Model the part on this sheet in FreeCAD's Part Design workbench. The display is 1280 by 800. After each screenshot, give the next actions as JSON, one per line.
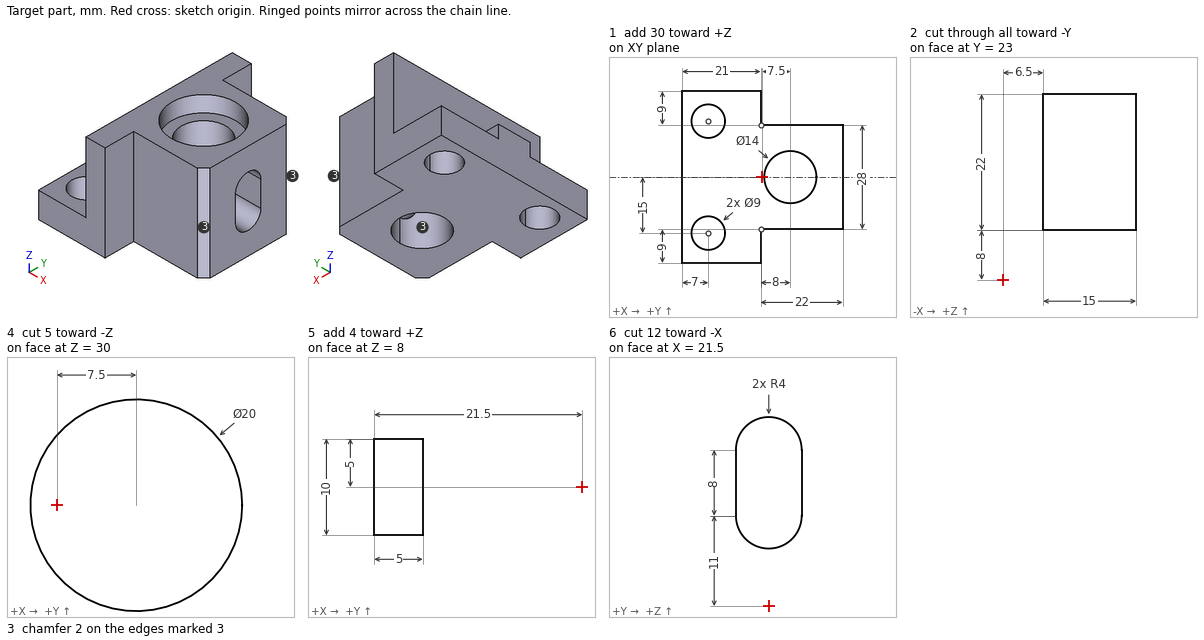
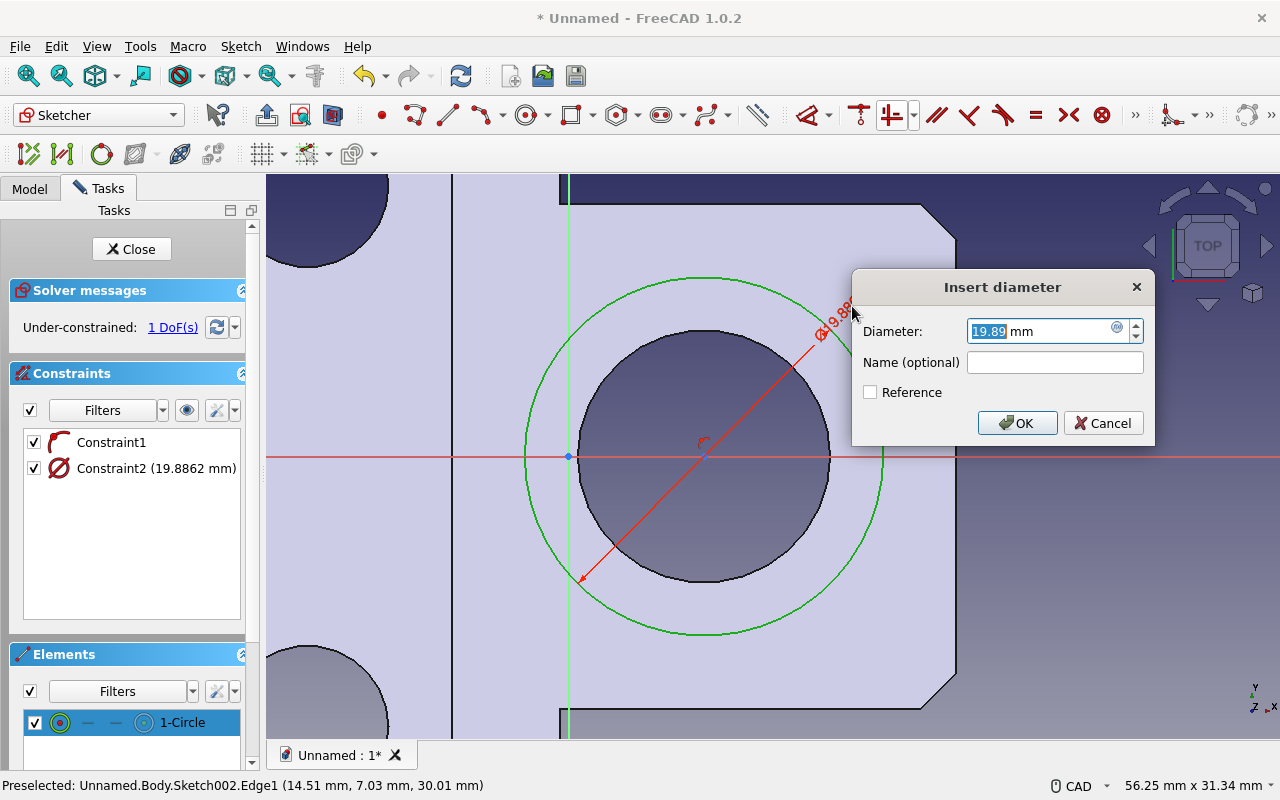
{"action": "type", "text": "20"}
{"action": "key", "text": "Return"}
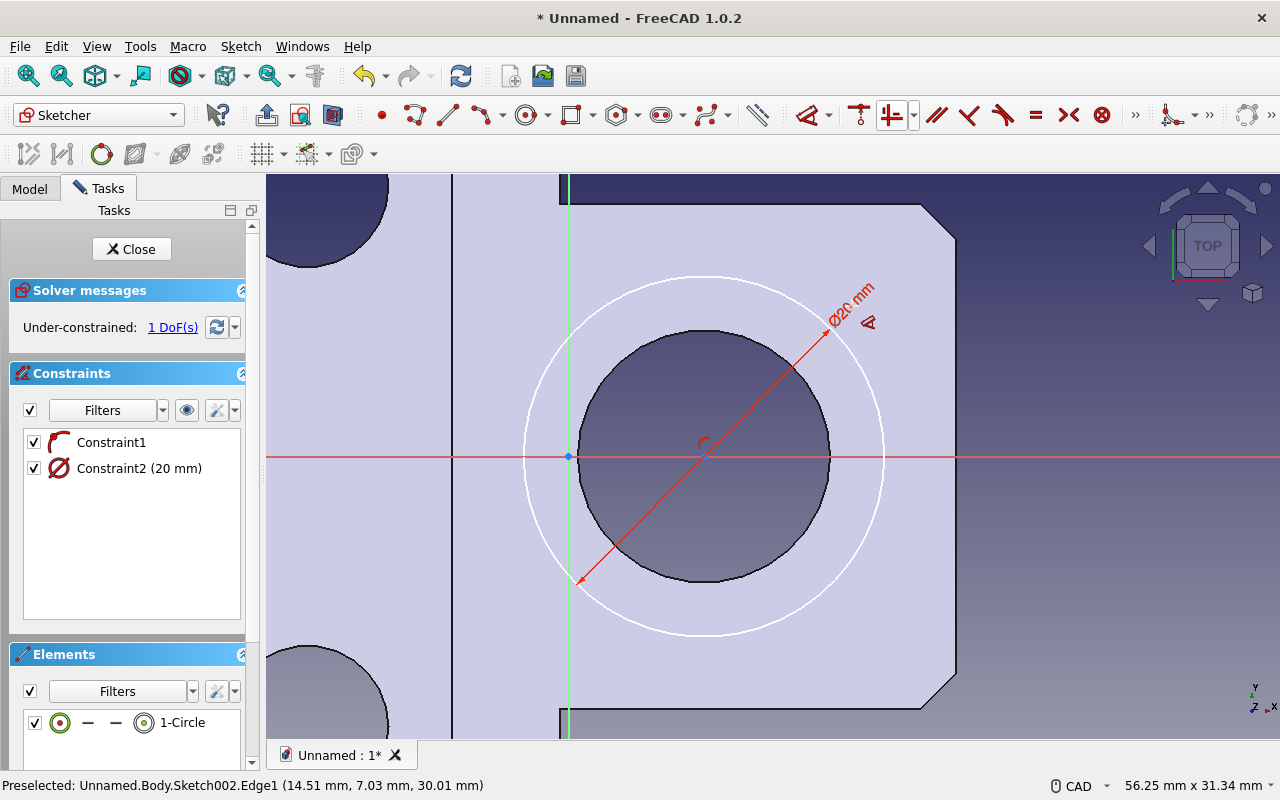
{"action": "left_click", "coordinate": [704, 456]}
{"action": "left_click", "coordinate": [636, 490]}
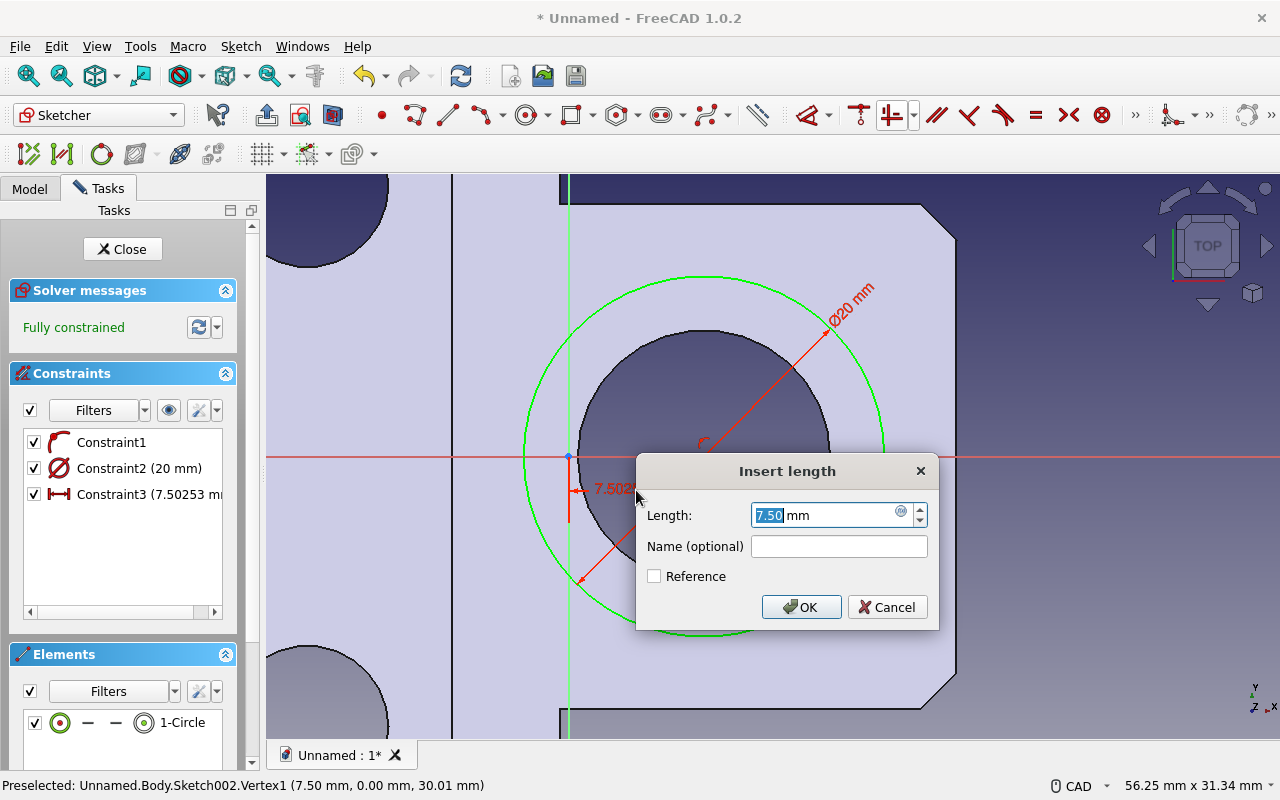
{"action": "type", "text": "7.5"}
{"action": "key", "text": "Return"}
{"action": "key", "text": "Escape"}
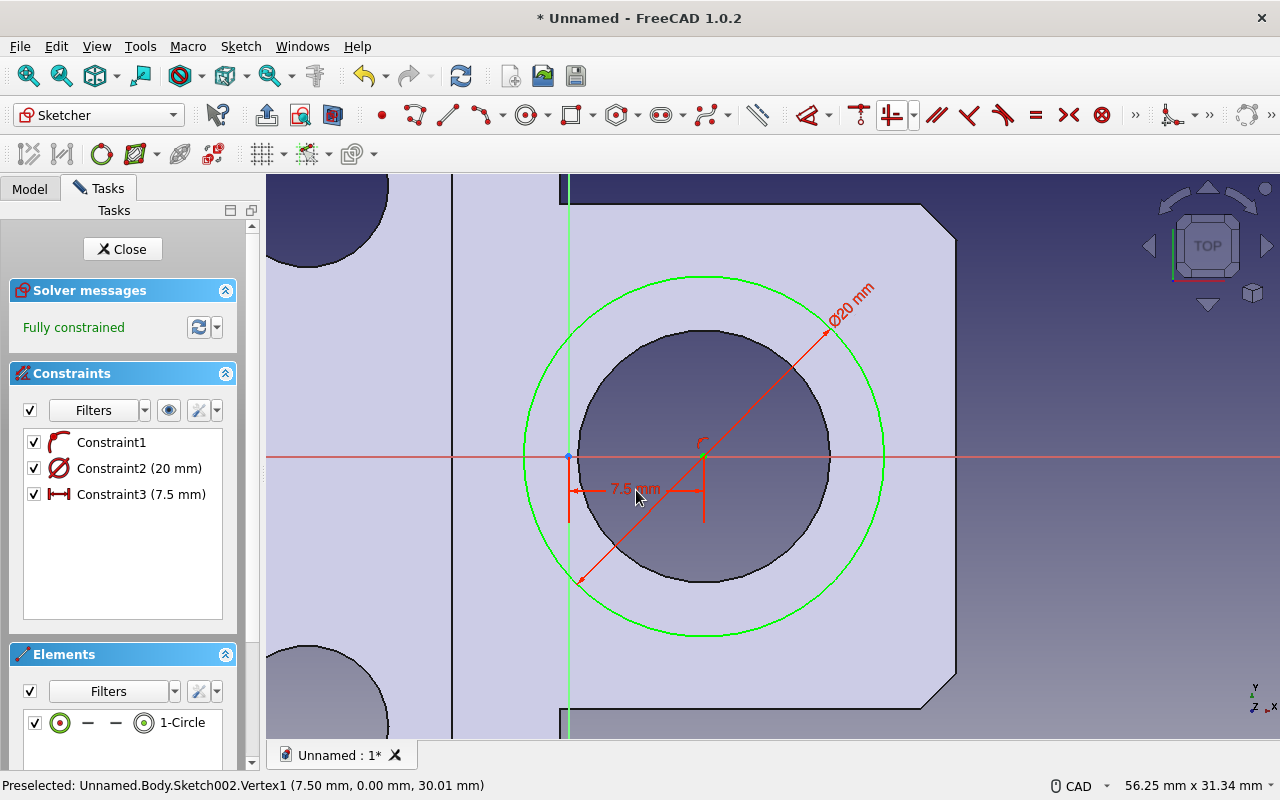
{"action": "left_click", "coordinate": [123, 249]}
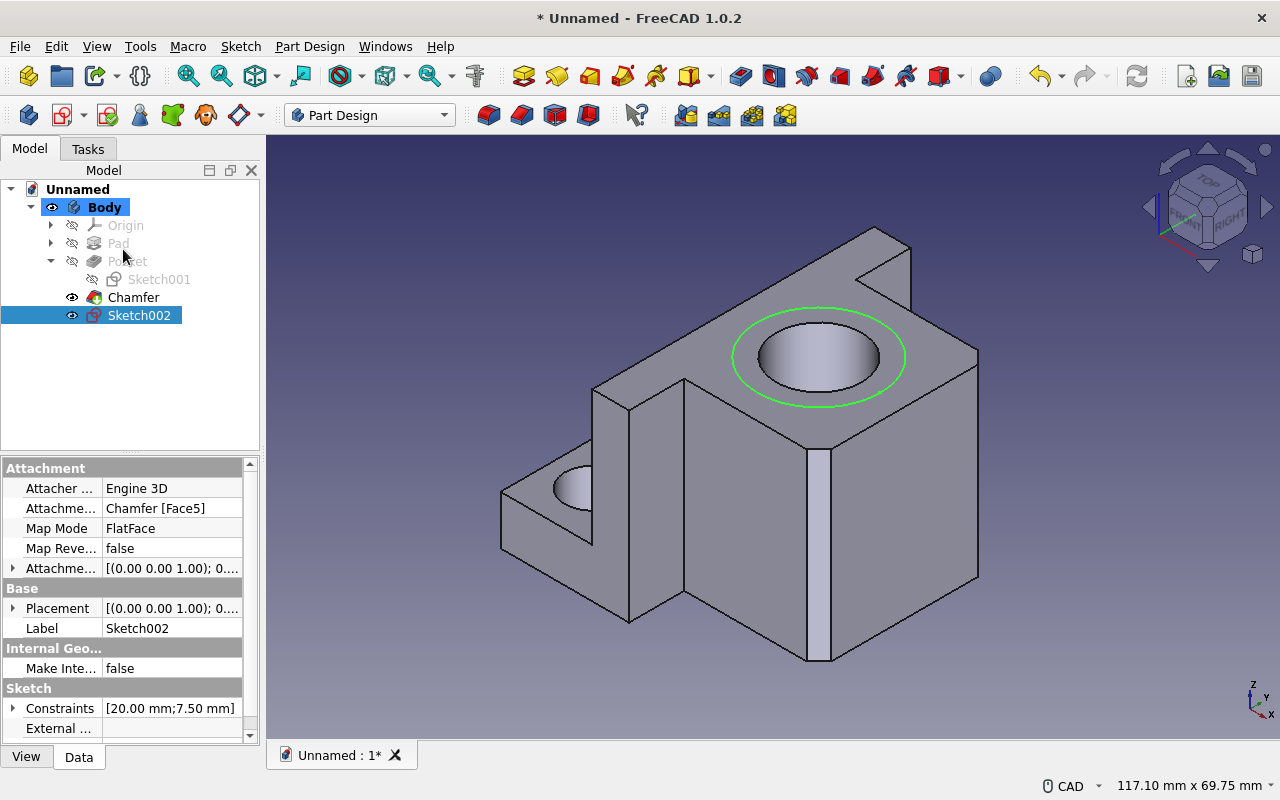
{"action": "left_click", "coordinate": [741, 76]}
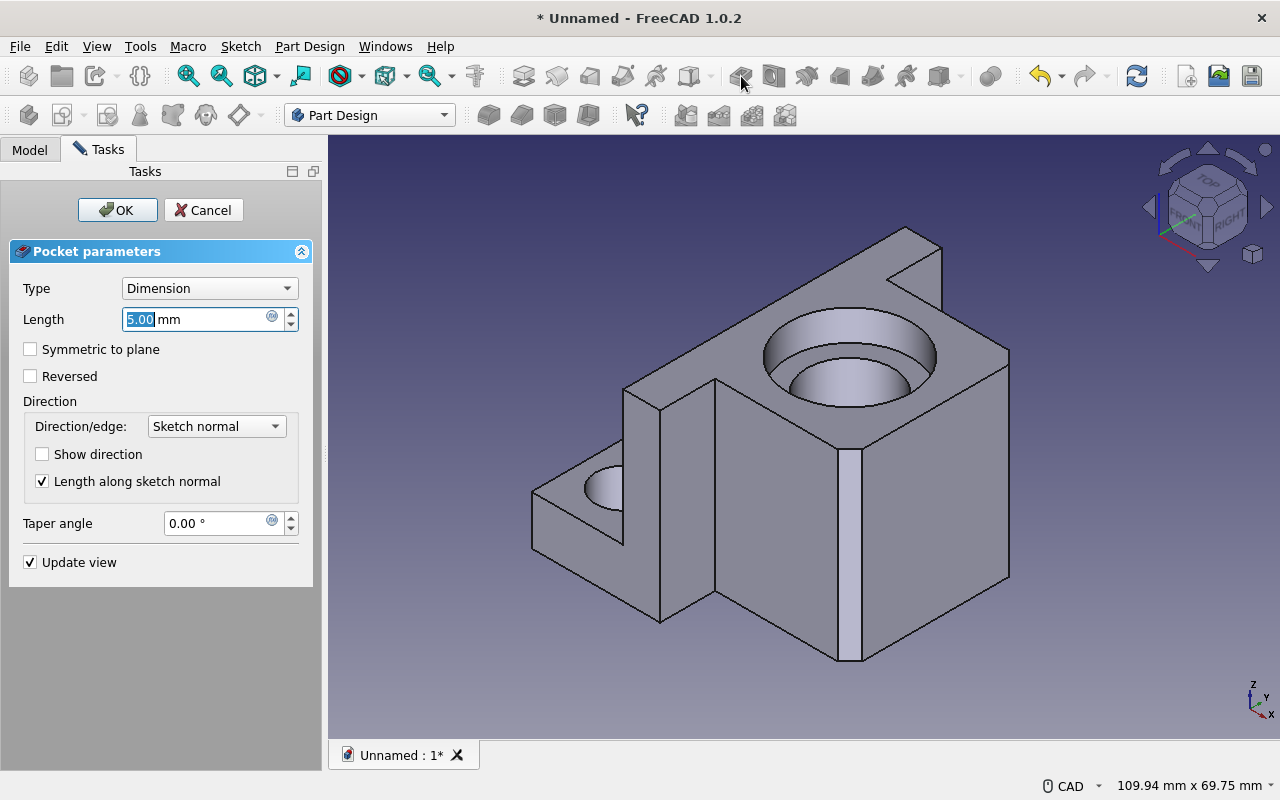
{"action": "type", "text": "5"}
{"action": "key", "text": "Tab"}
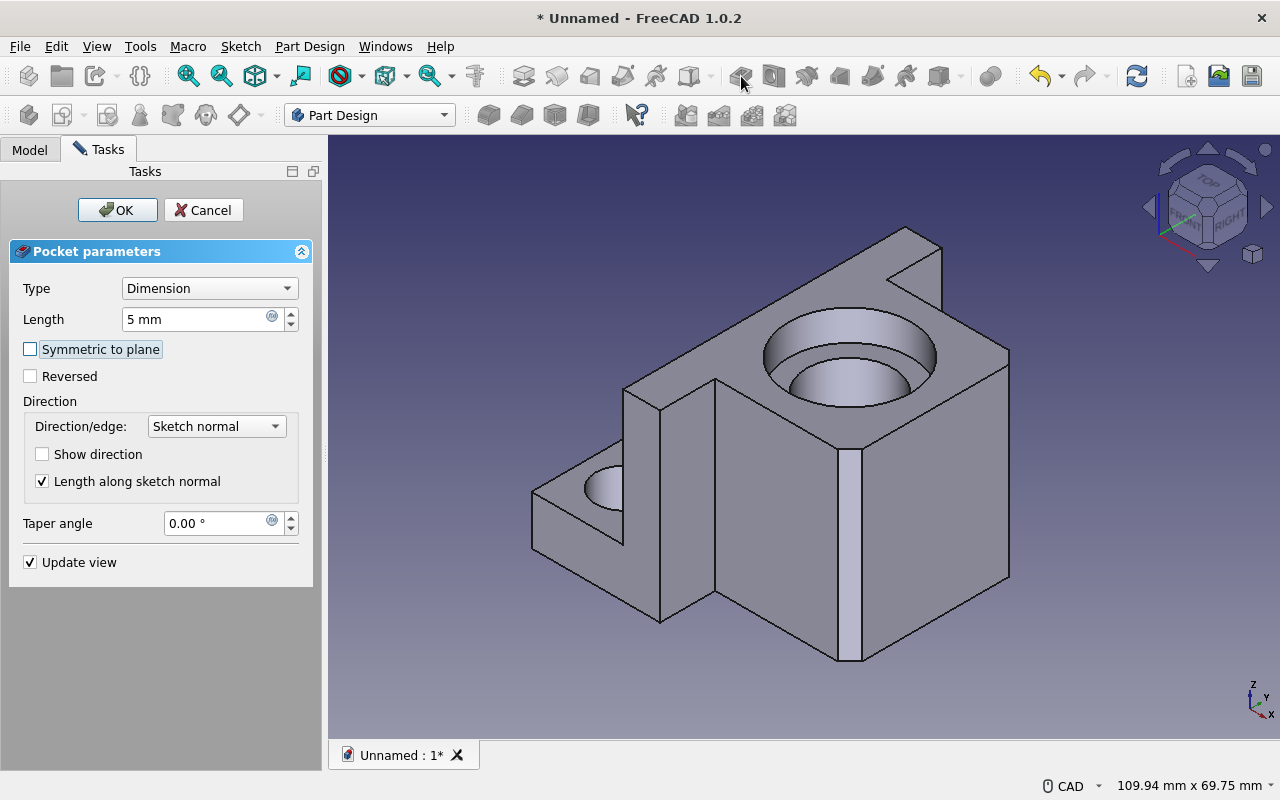
{"action": "left_click", "coordinate": [118, 210]}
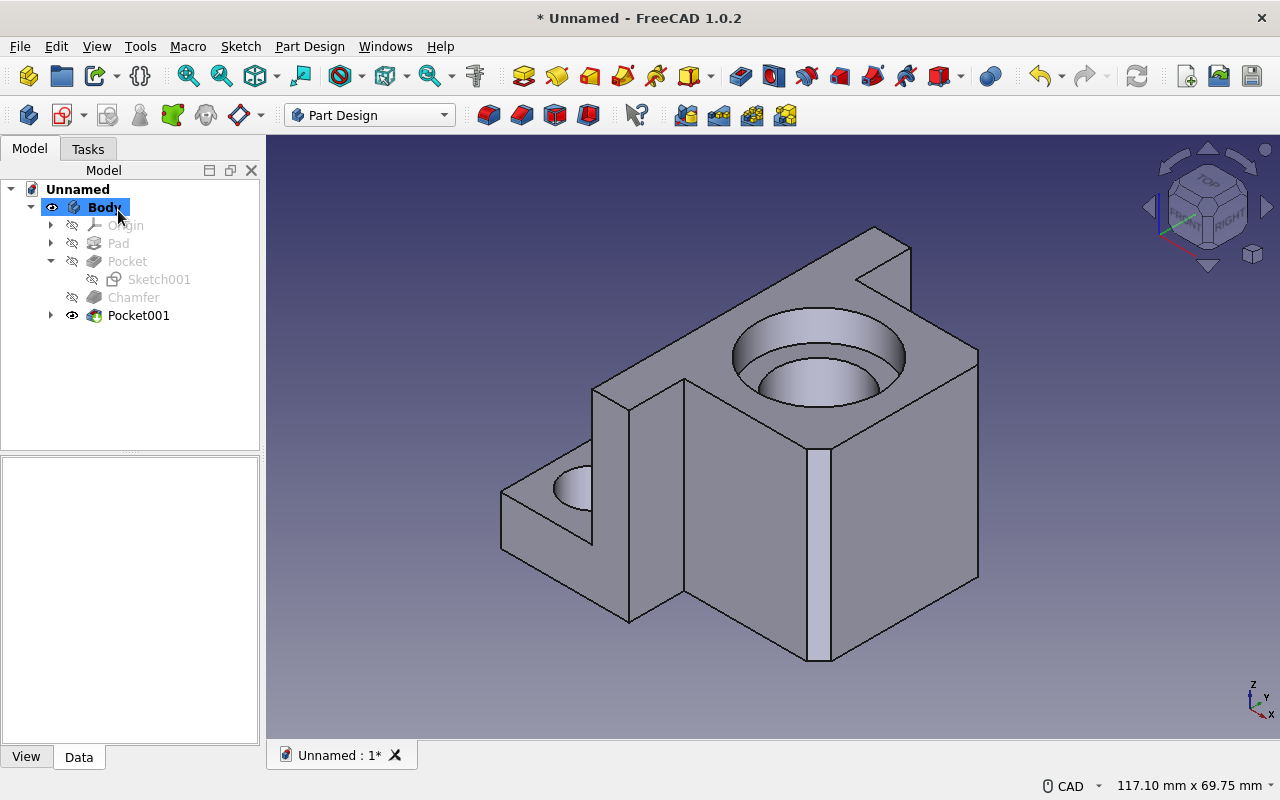
{"action": "key", "text": "2"}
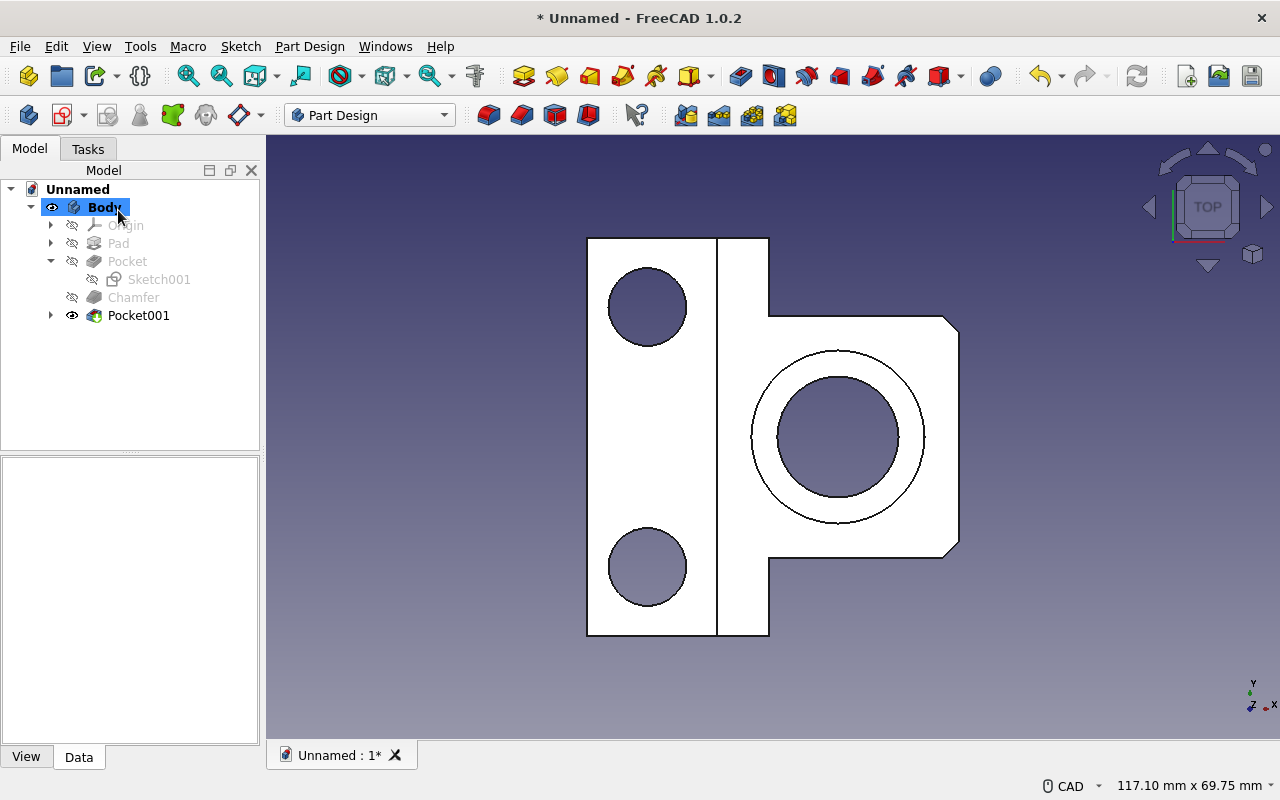
{"action": "left_click", "coordinate": [652, 436]}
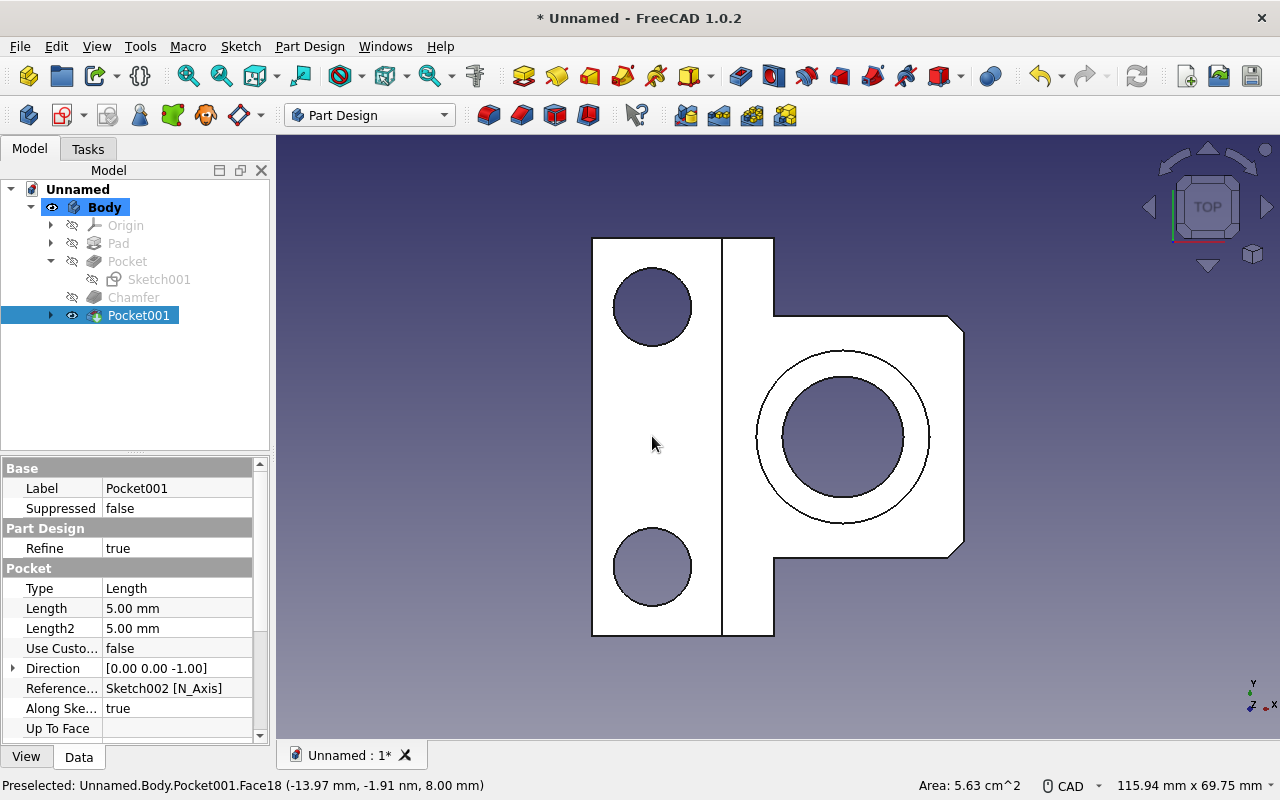
{"action": "left_click", "coordinate": [62, 116]}